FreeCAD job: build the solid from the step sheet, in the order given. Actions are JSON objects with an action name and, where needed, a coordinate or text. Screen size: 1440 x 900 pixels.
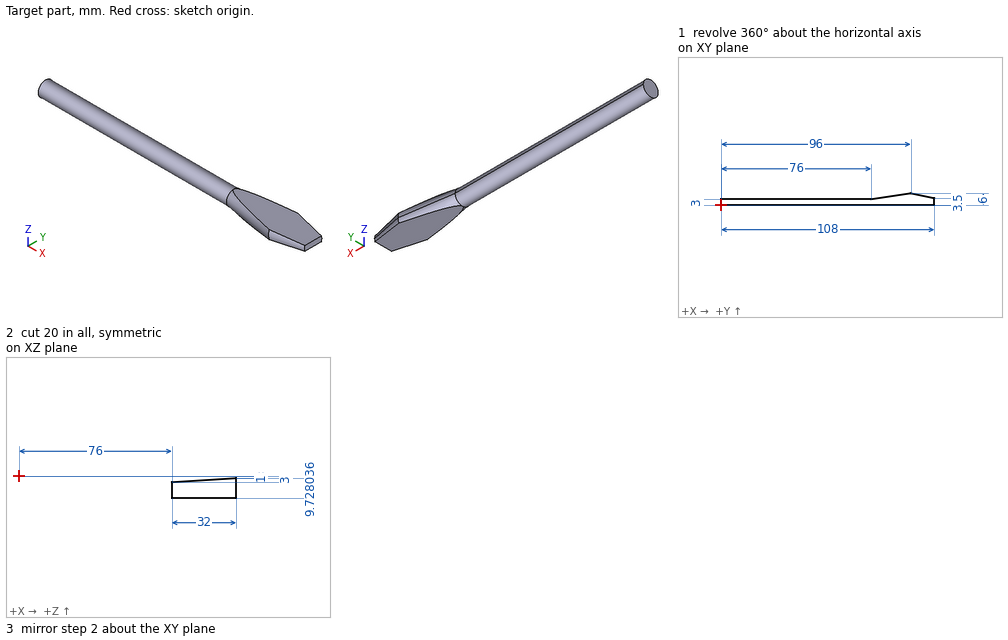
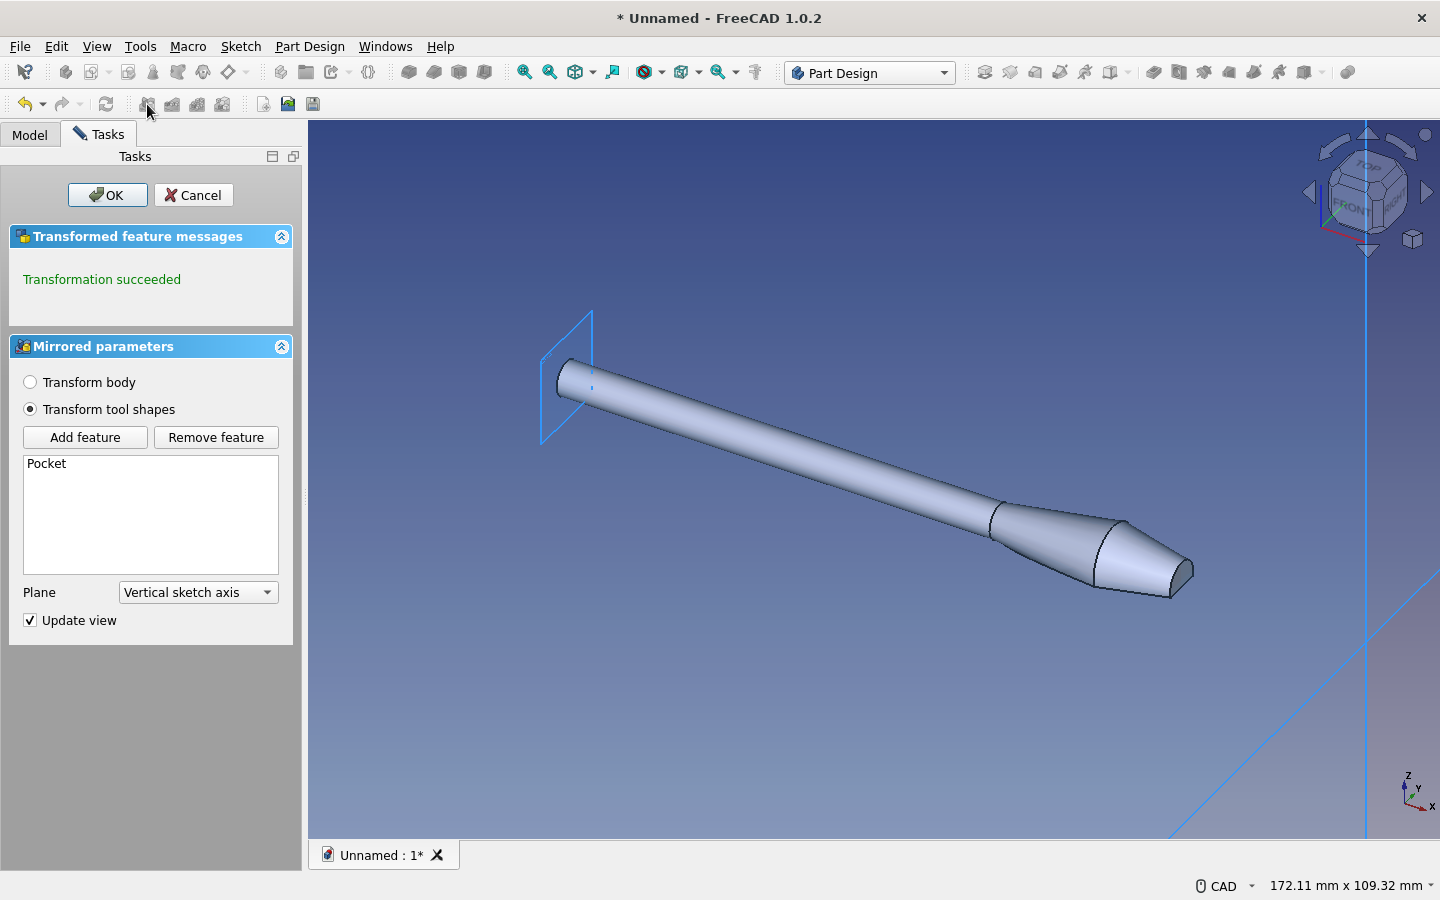
{"action": "left_click", "coordinate": [199, 592]}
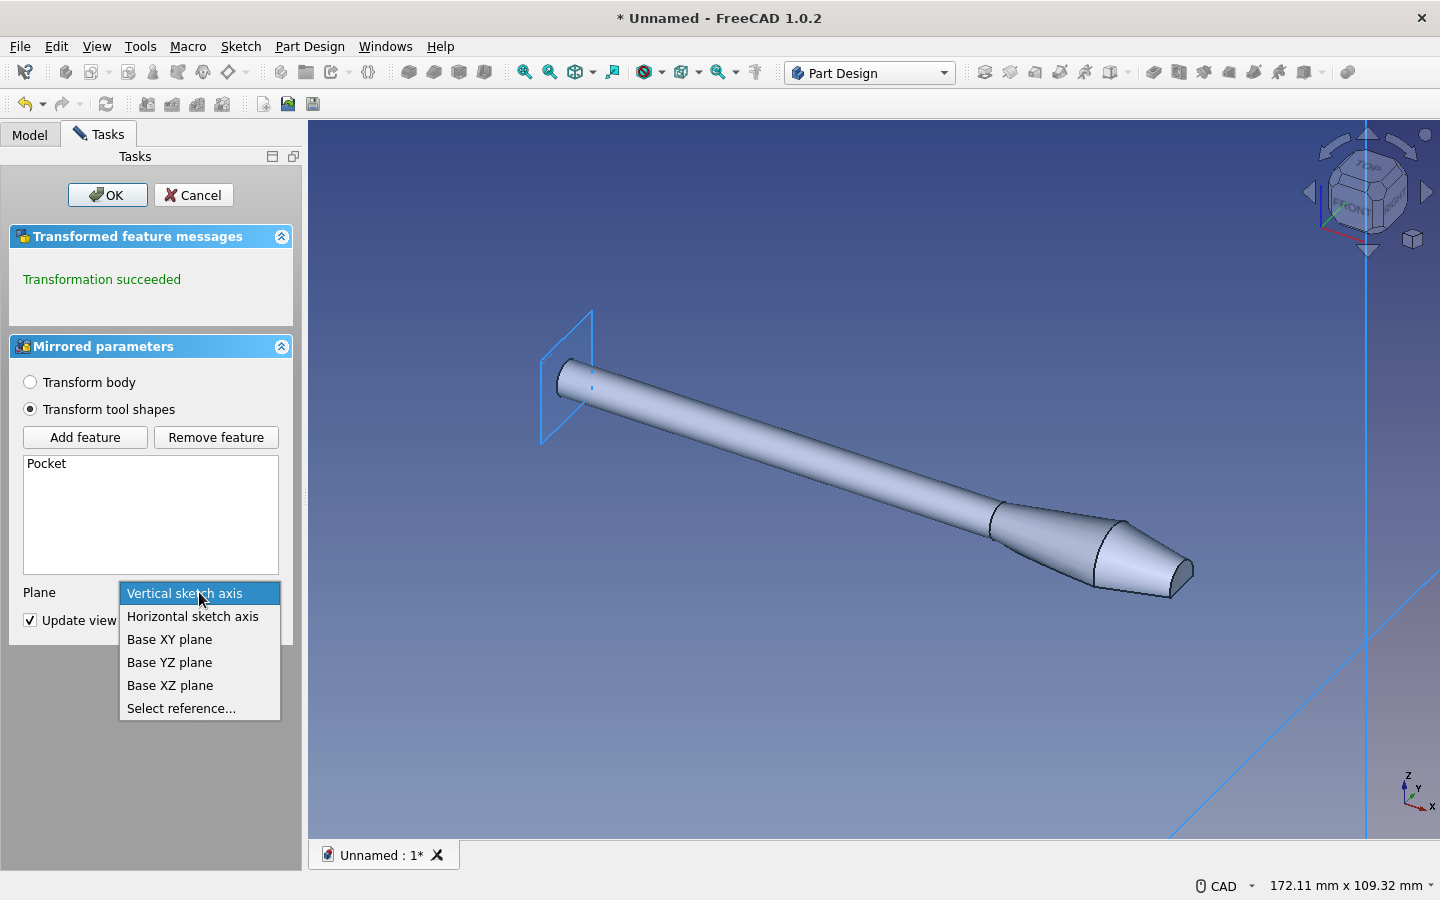
{"action": "left_click", "coordinate": [198, 640]}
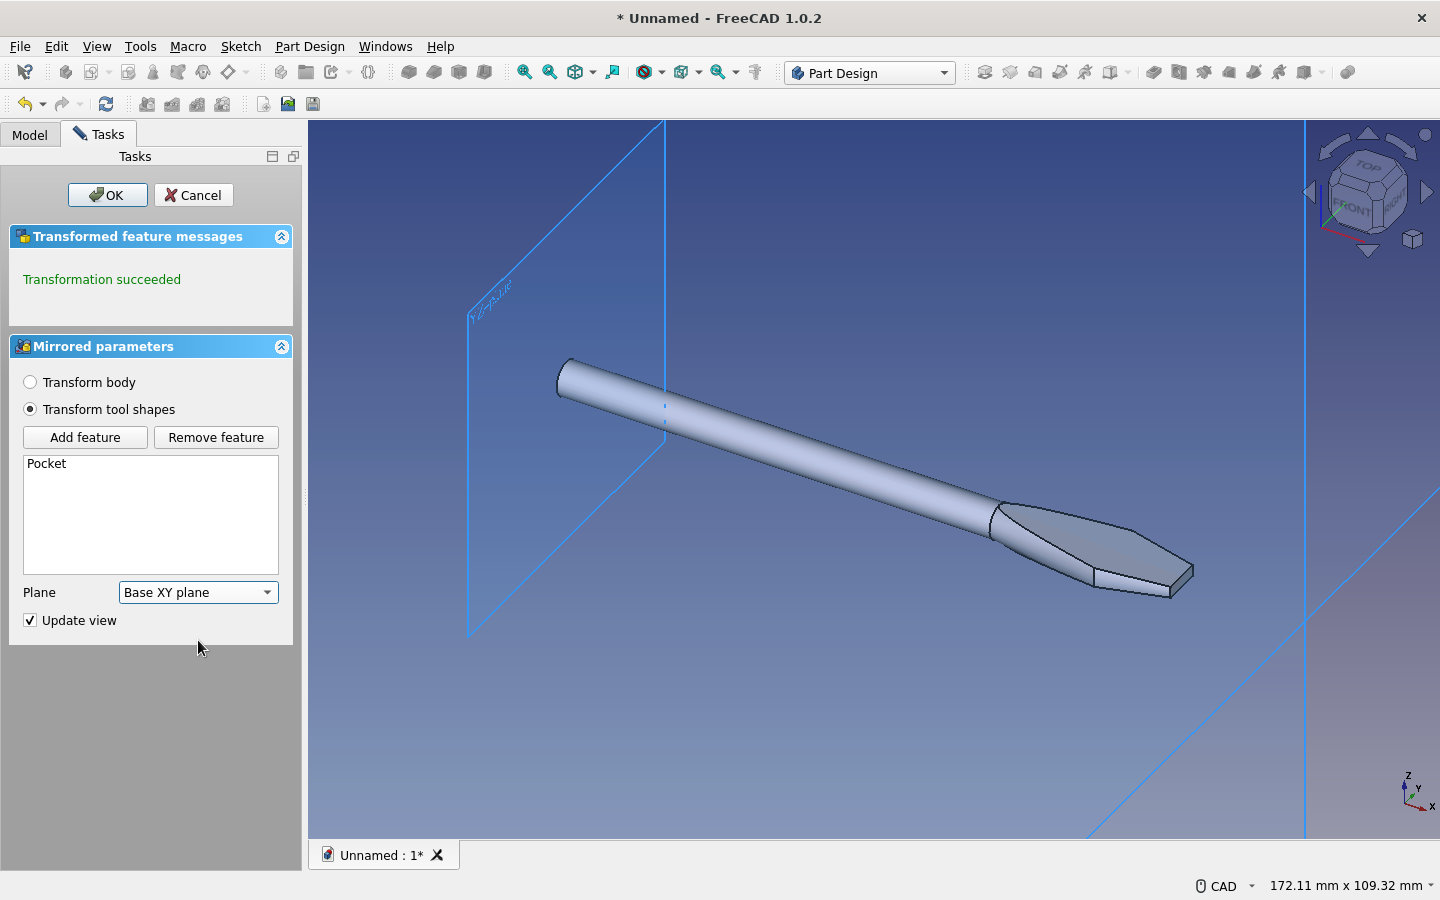
{"action": "left_click", "coordinate": [108, 195]}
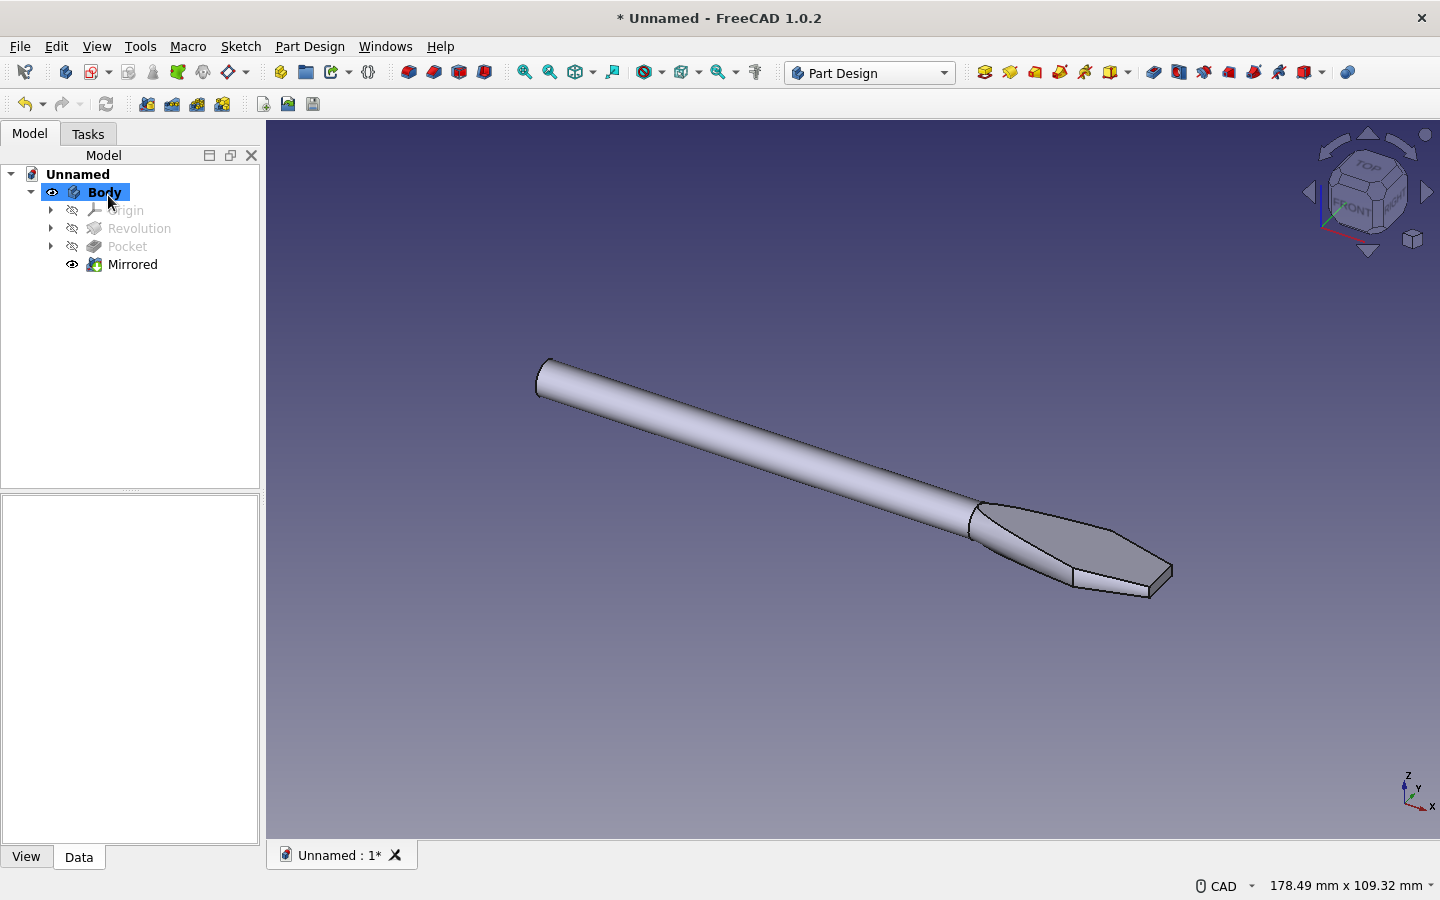
{"action": "key", "text": "0"}